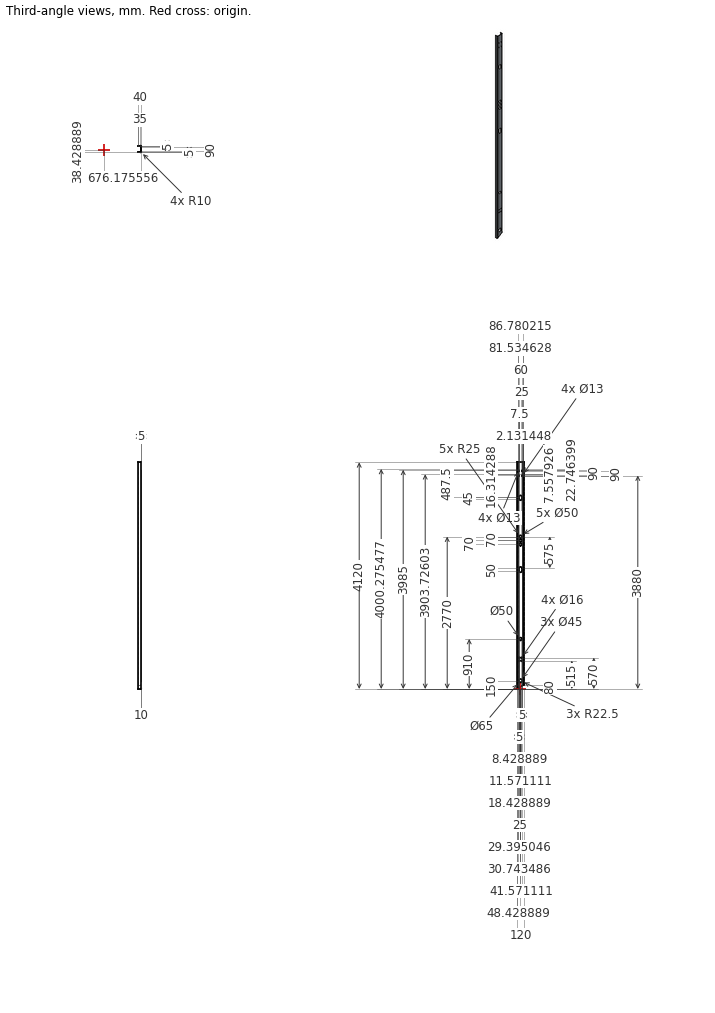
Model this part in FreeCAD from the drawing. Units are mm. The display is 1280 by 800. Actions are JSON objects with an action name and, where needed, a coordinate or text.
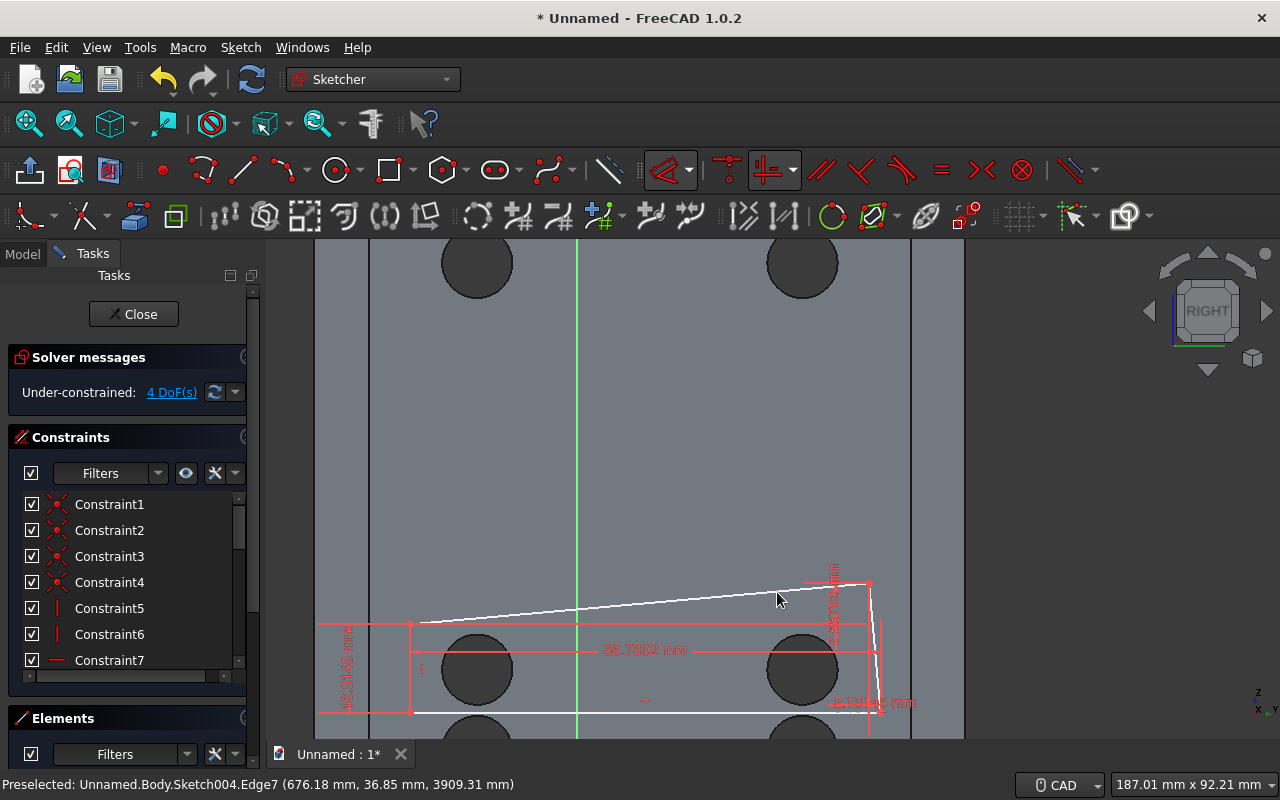
{"action": "scroll", "coordinate": [776, 591], "scroll_direction": "down", "scroll_amount": 3}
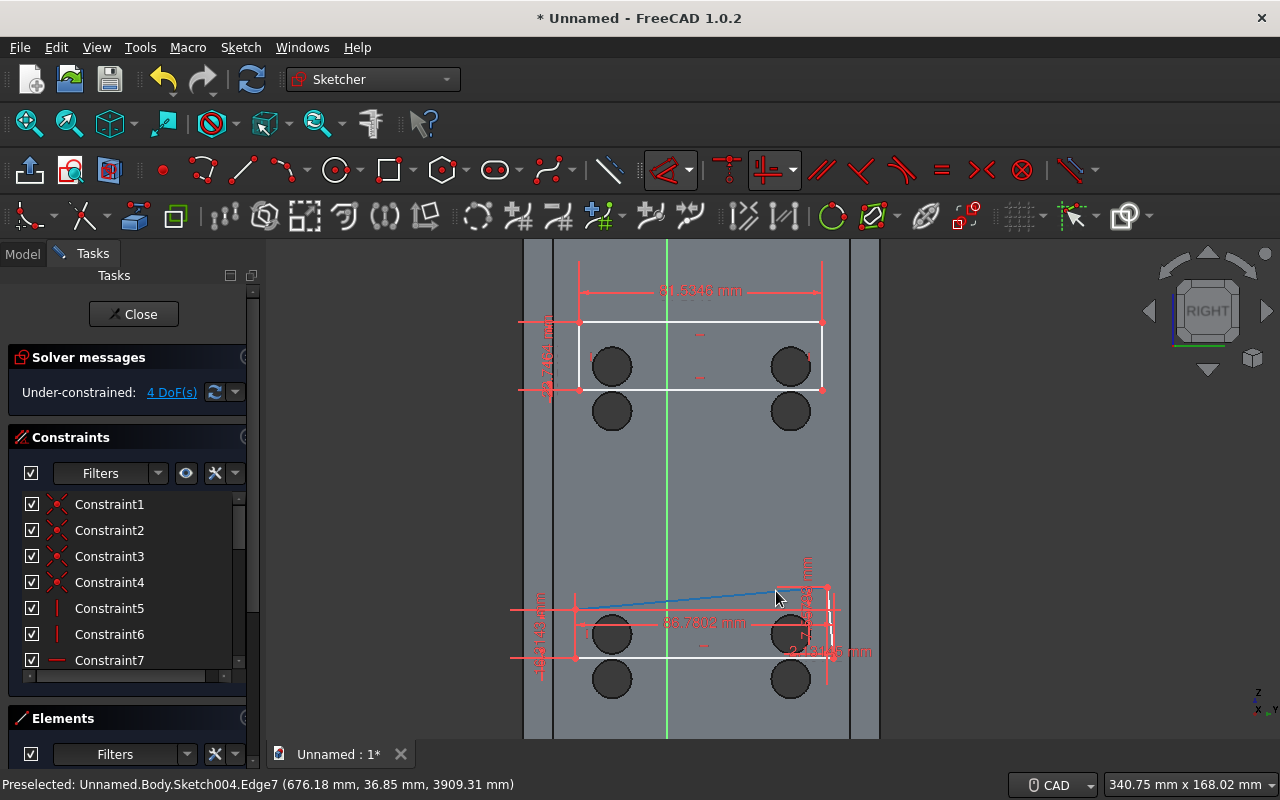
{"action": "left_click", "coordinate": [579, 322]}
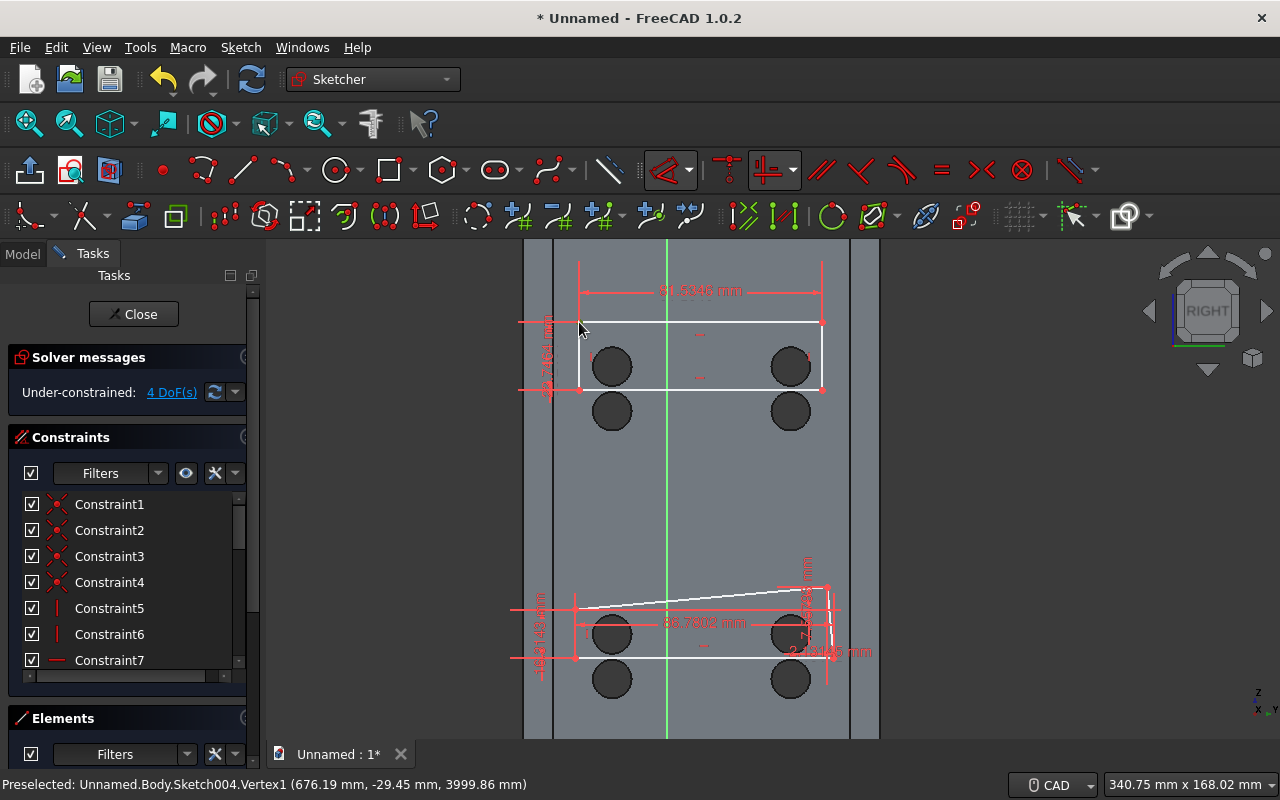
{"action": "key", "text": "l"}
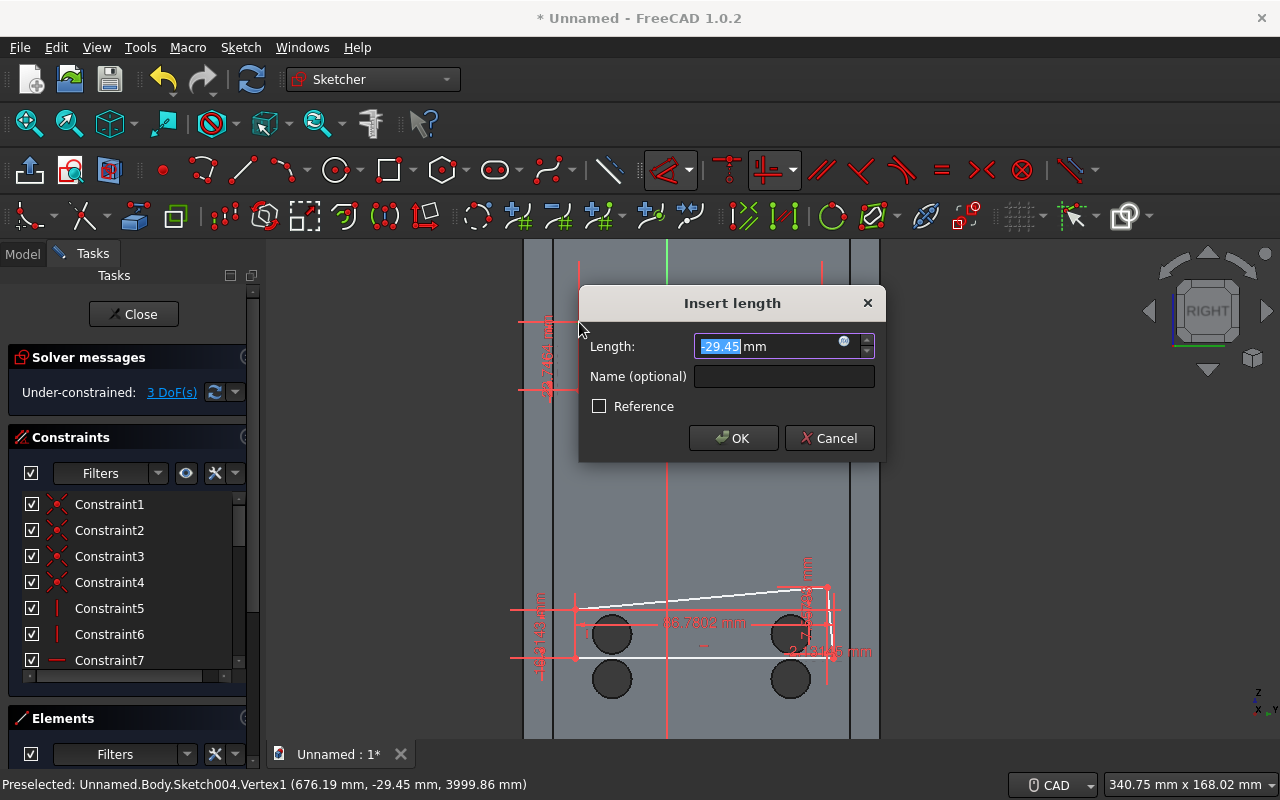
{"action": "type", "text": "-29.395046"}
{"action": "key", "text": "Return"}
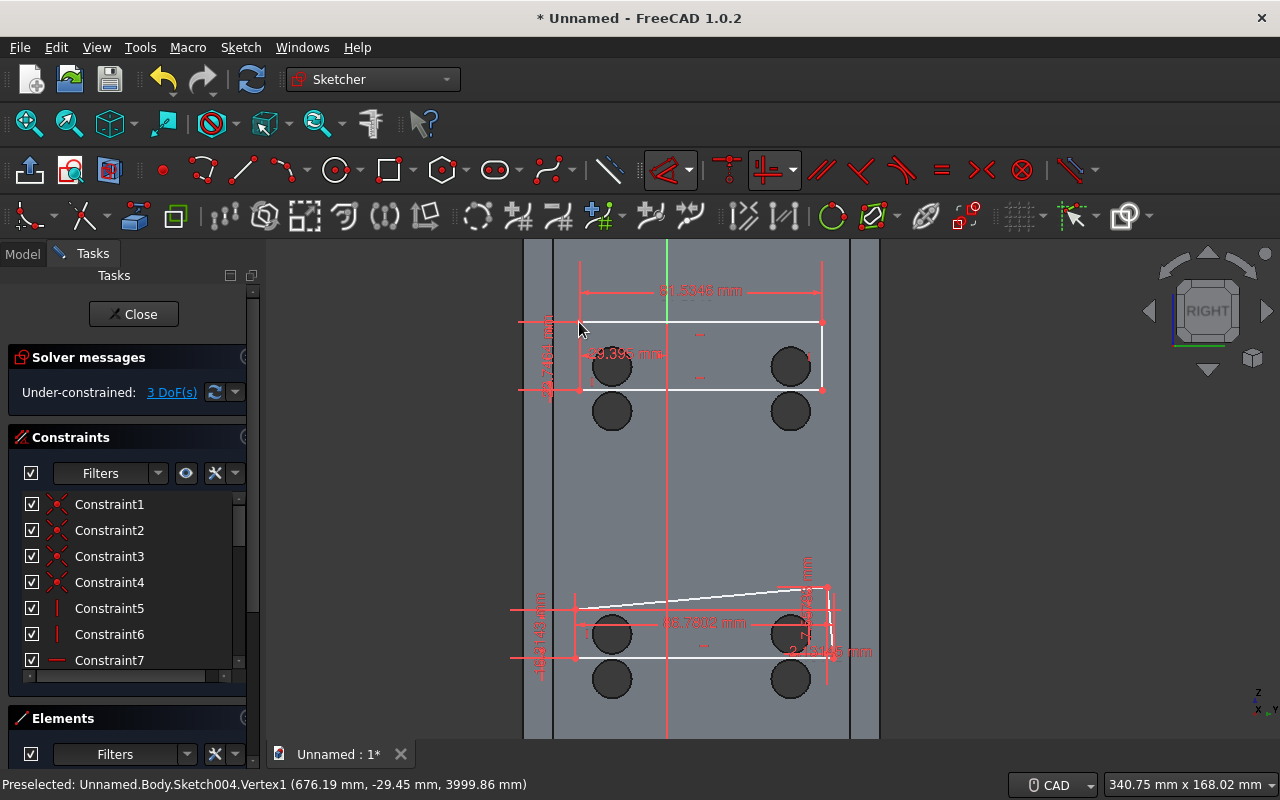
{"action": "left_click", "coordinate": [575, 658]}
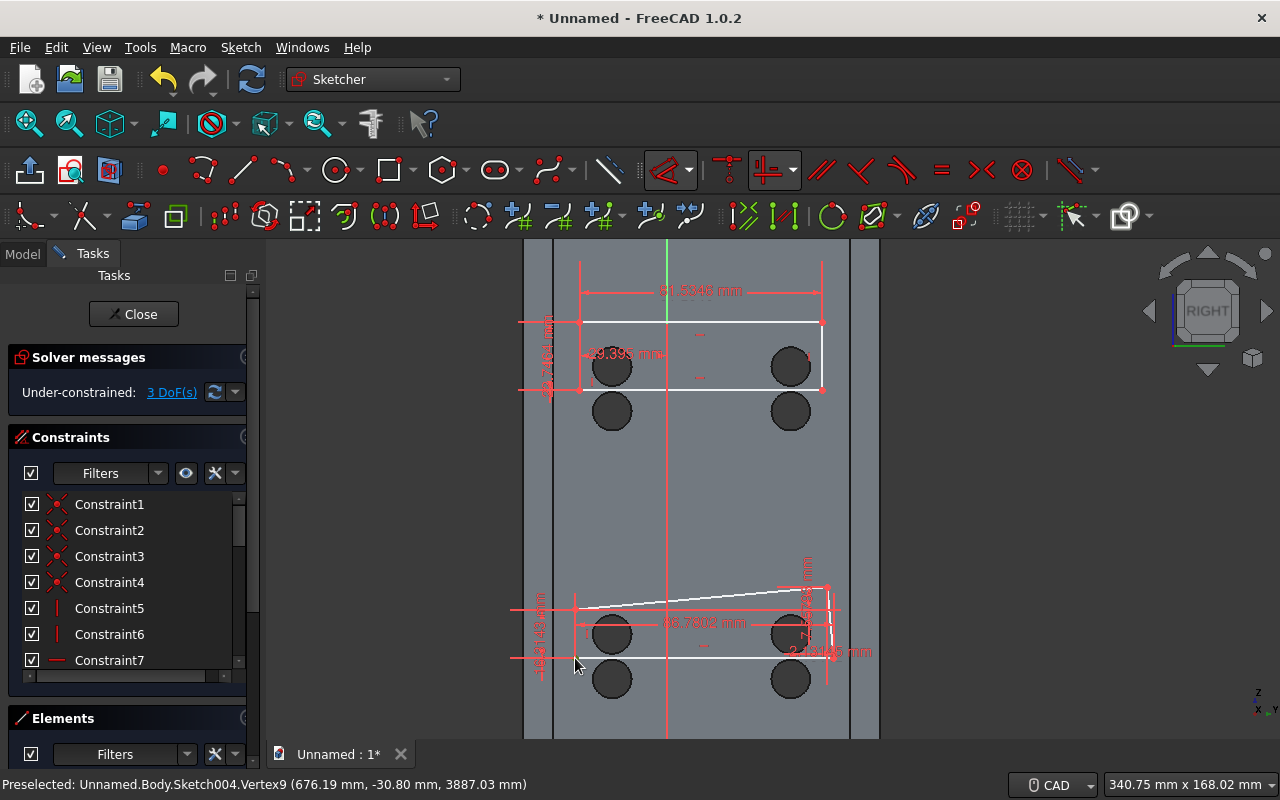
{"action": "left_click", "coordinate": [692, 170]}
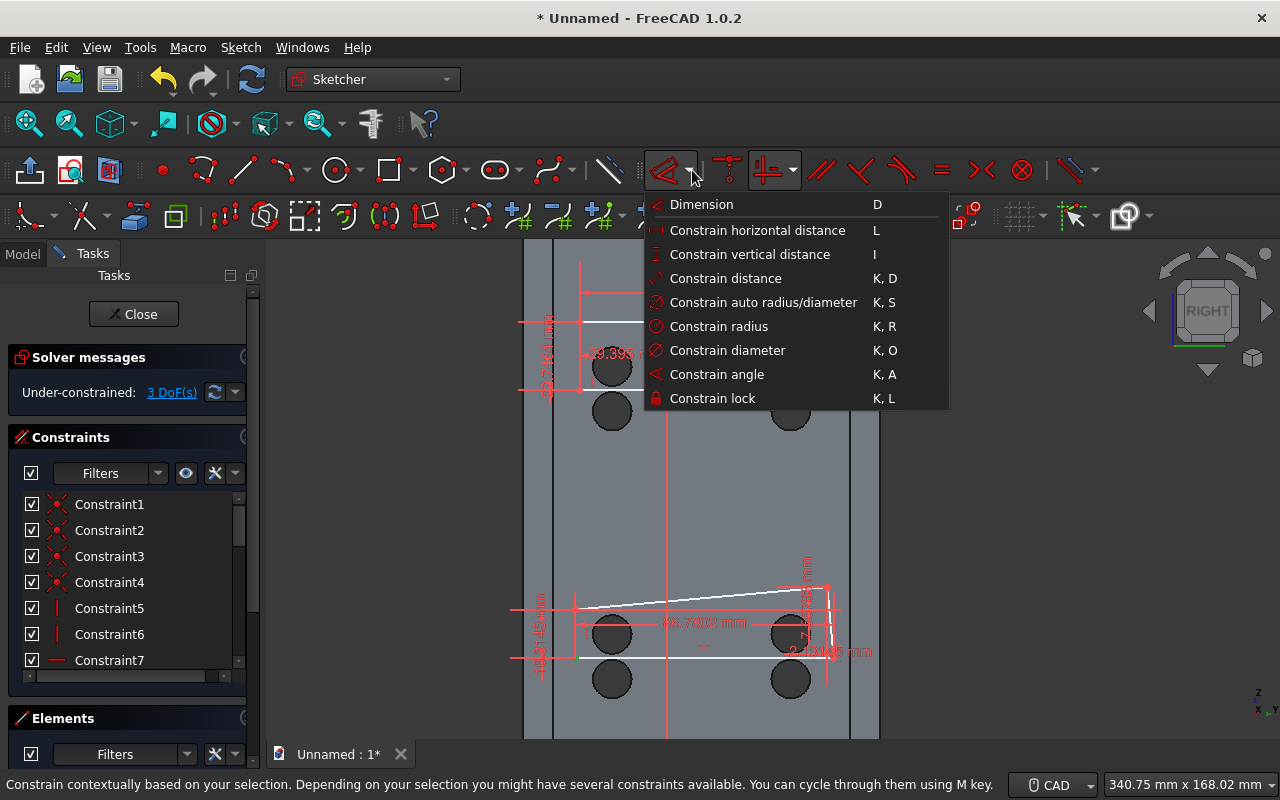
{"action": "left_click", "coordinate": [797, 230]}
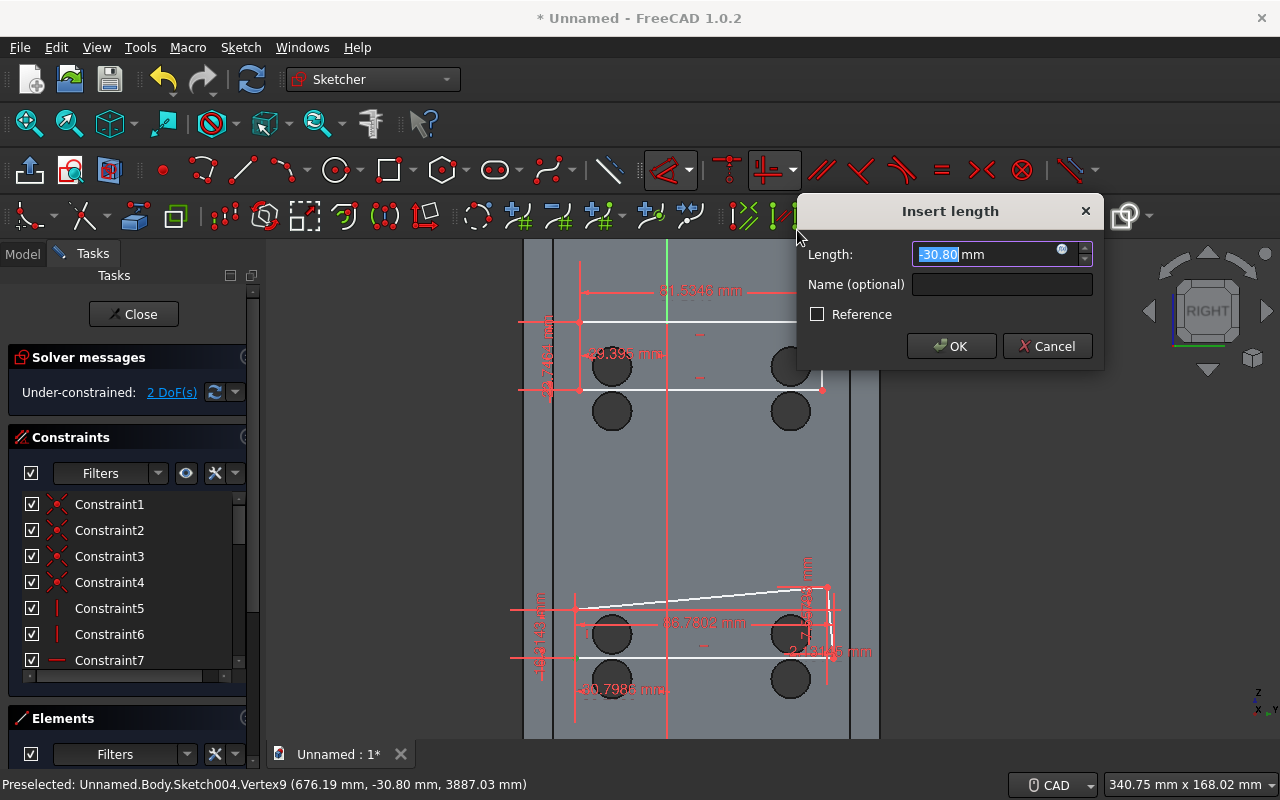
{"action": "type", "text": "-30.743486"}
{"action": "key", "text": "Return"}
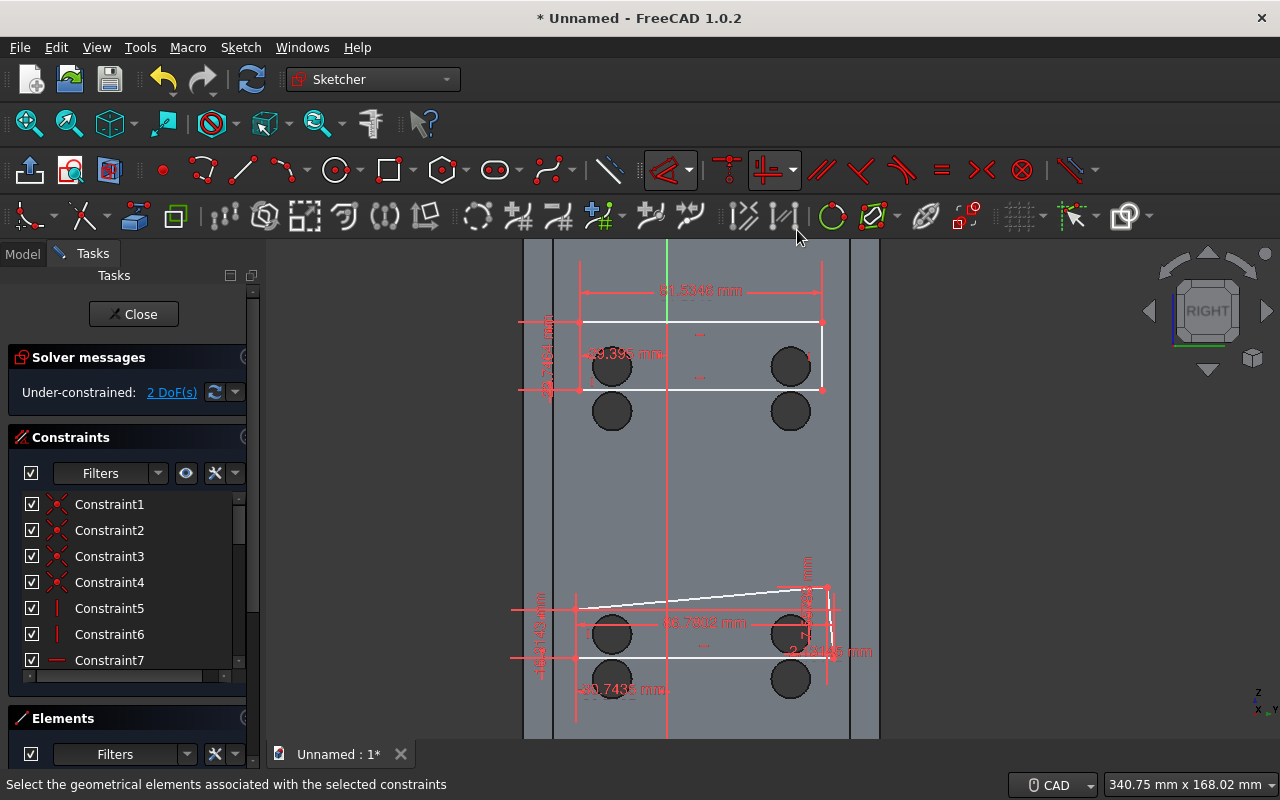
{"action": "left_click", "coordinate": [576, 610]}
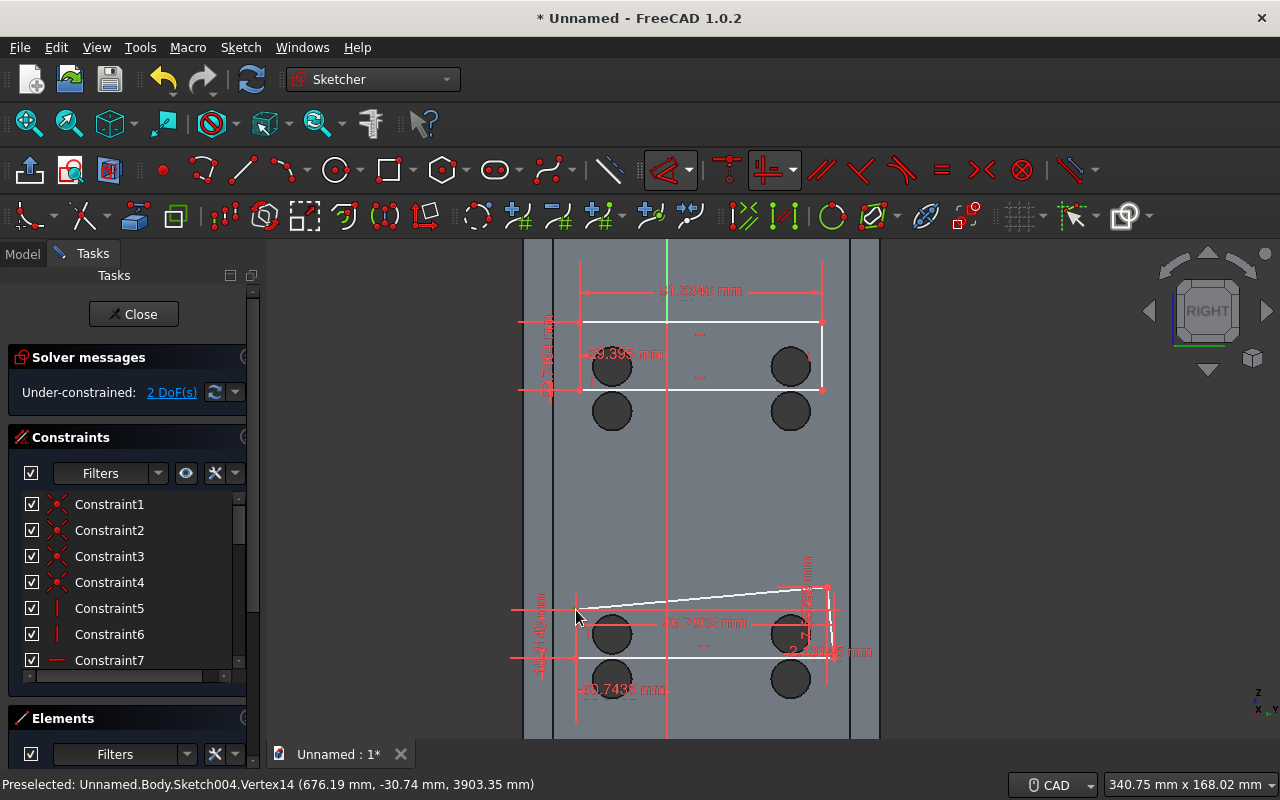
{"action": "key", "text": "i"}